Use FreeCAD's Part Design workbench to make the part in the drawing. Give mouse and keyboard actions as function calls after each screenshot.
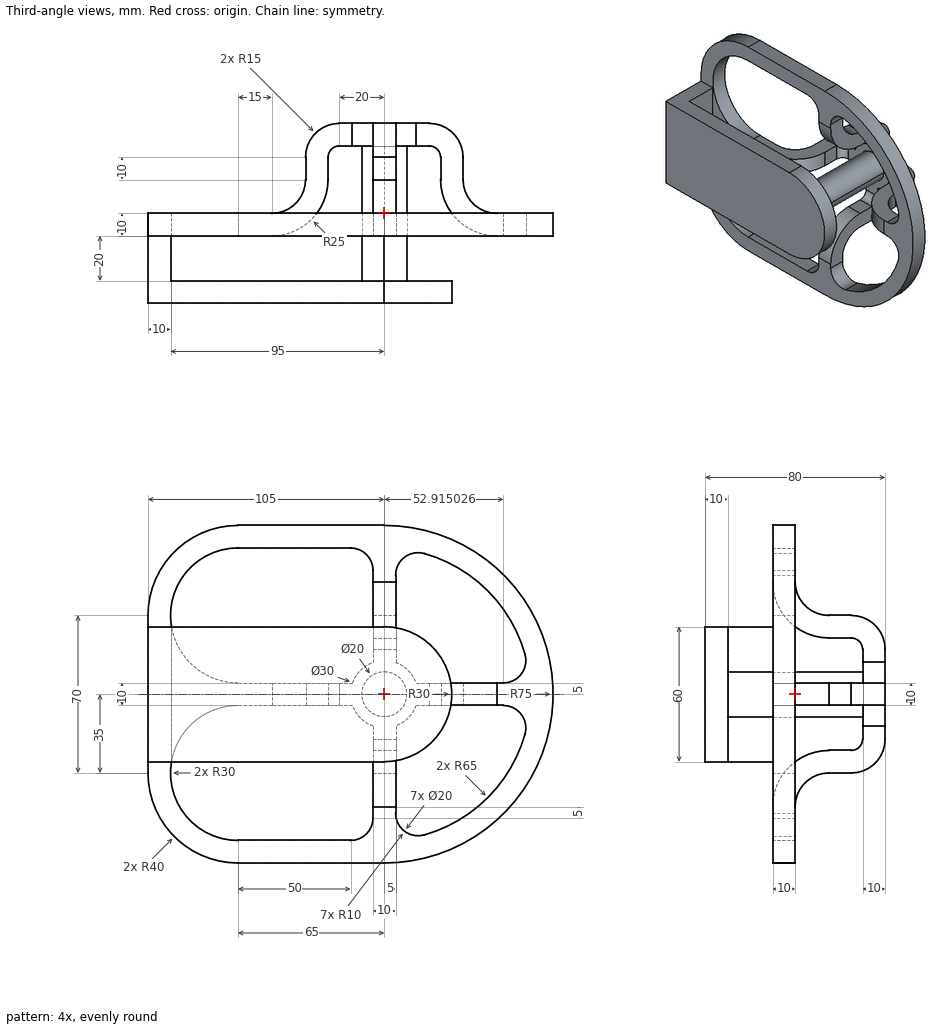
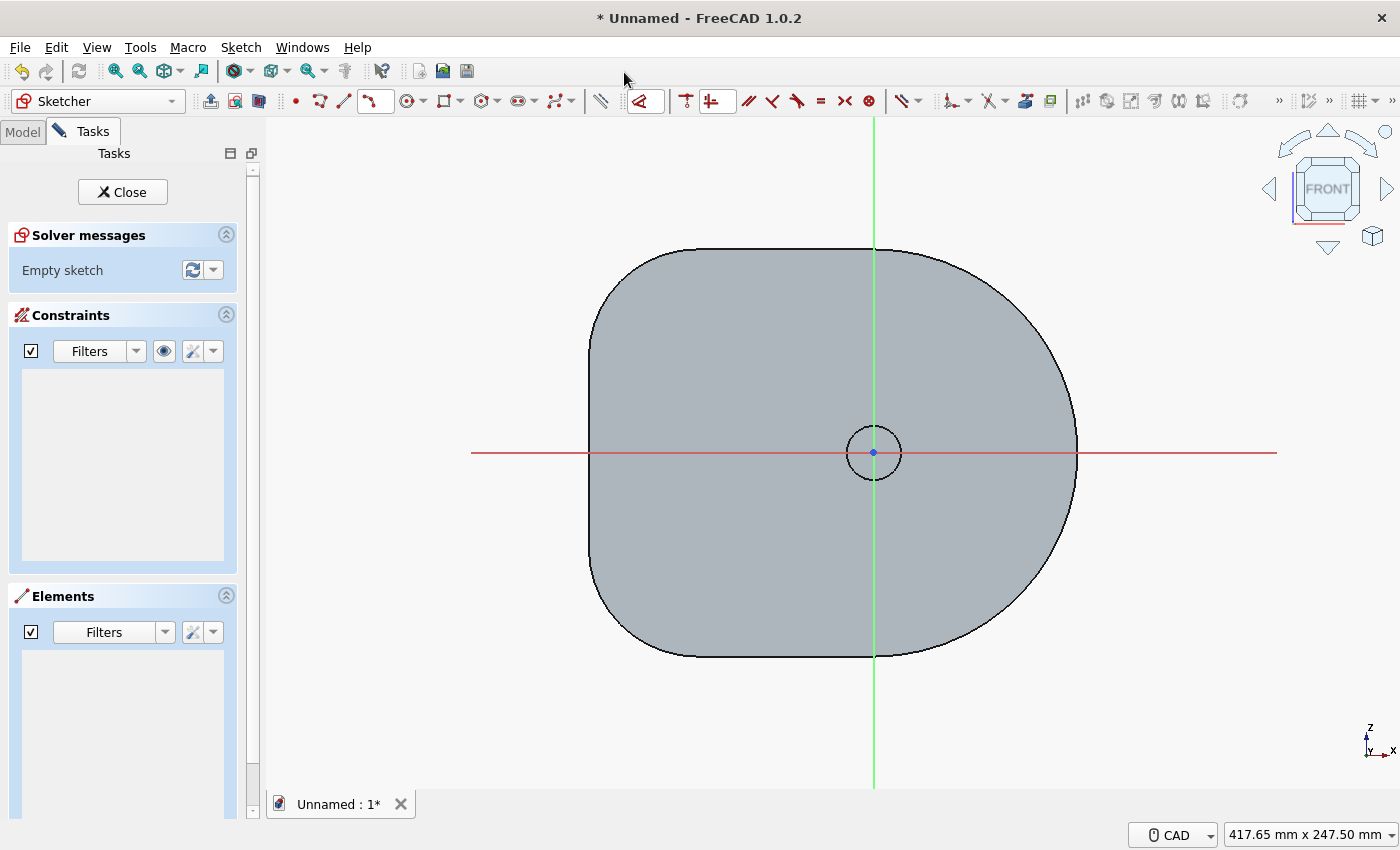
scroll(781, 453, up, 3)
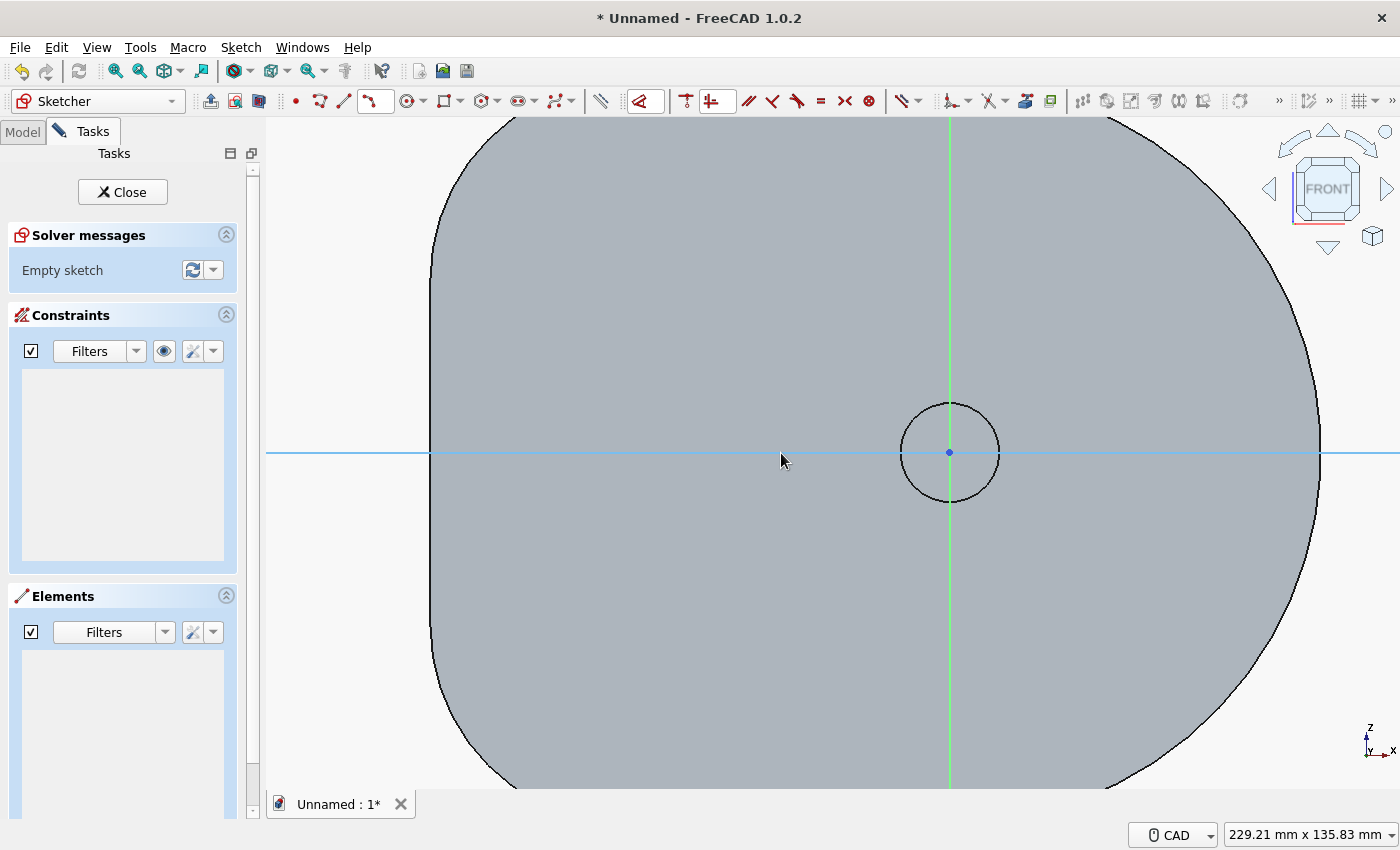
click(320, 102)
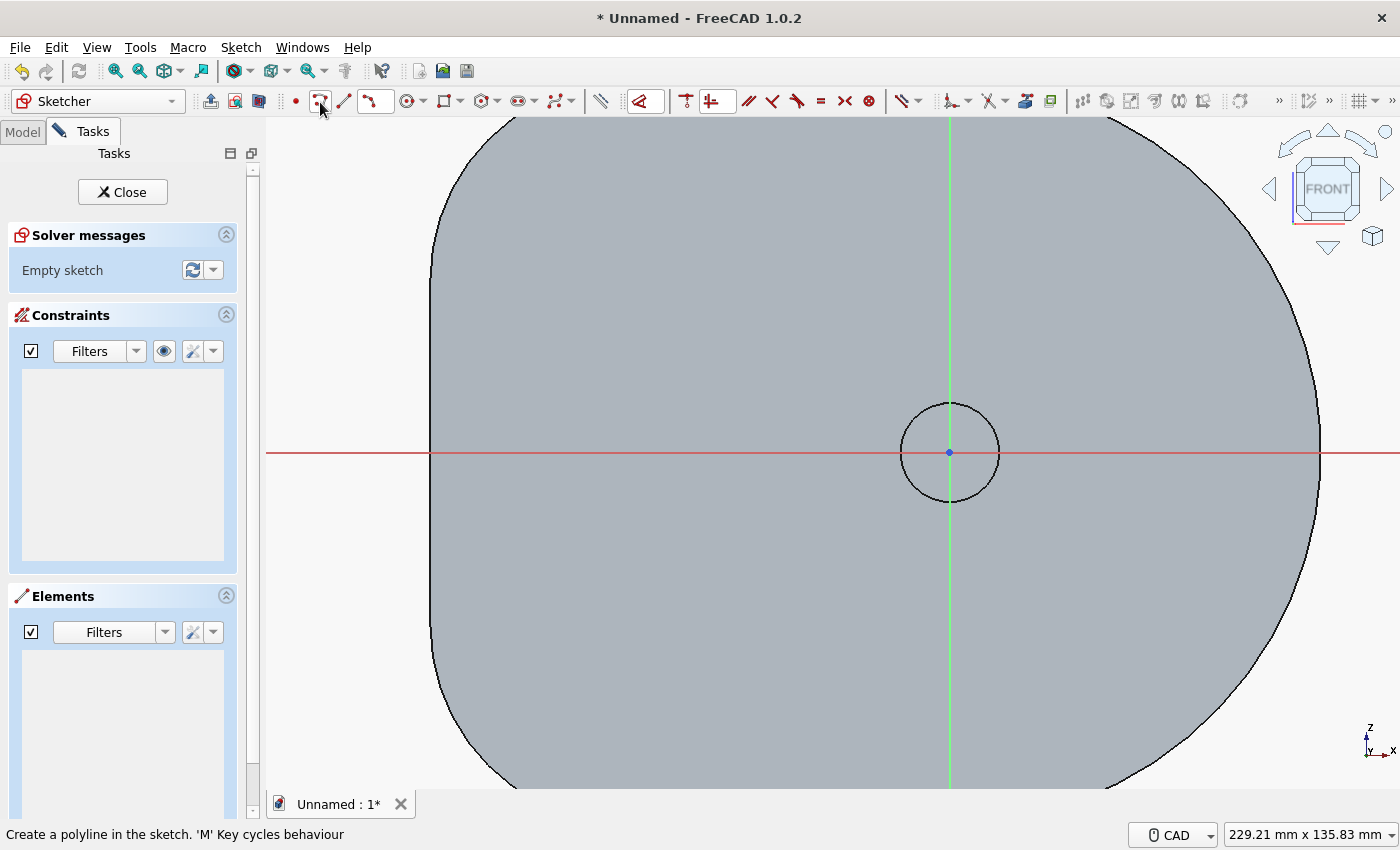
click(950, 304)
click(430, 304)
click(430, 601)
click(950, 601)
right_click(950, 601)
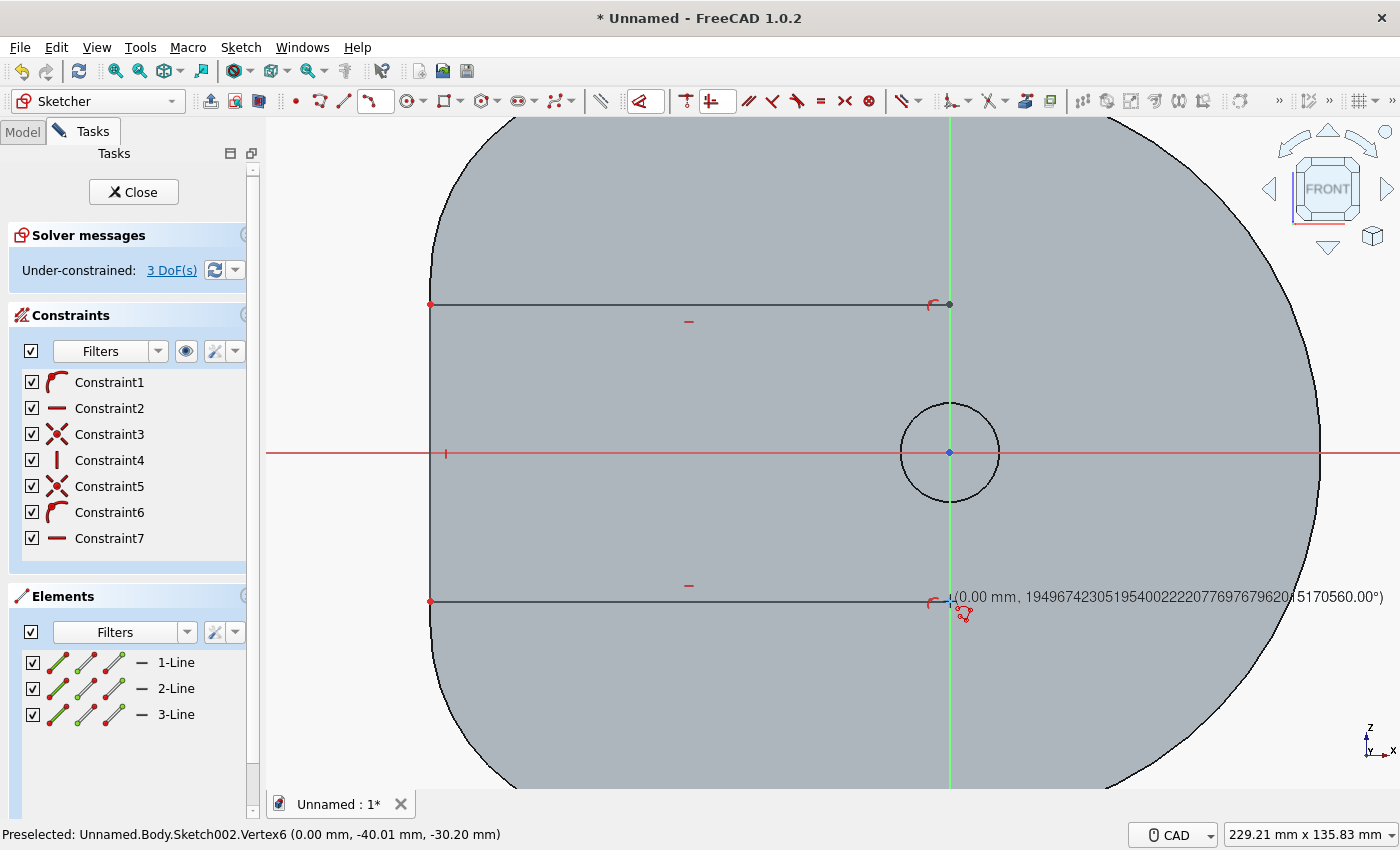
click(370, 102)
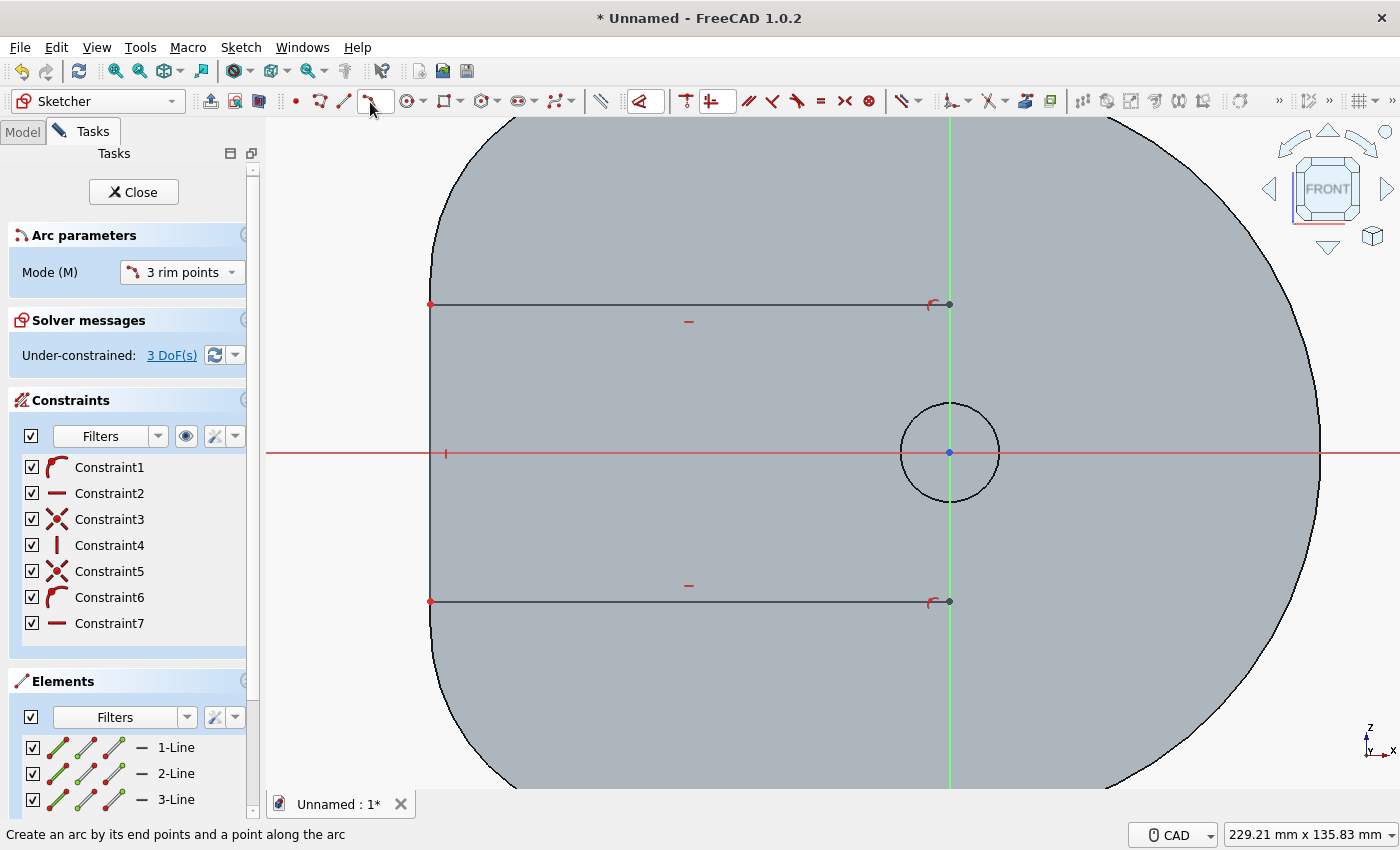
click(950, 602)
click(950, 305)
click(1091, 498)
key(Escape)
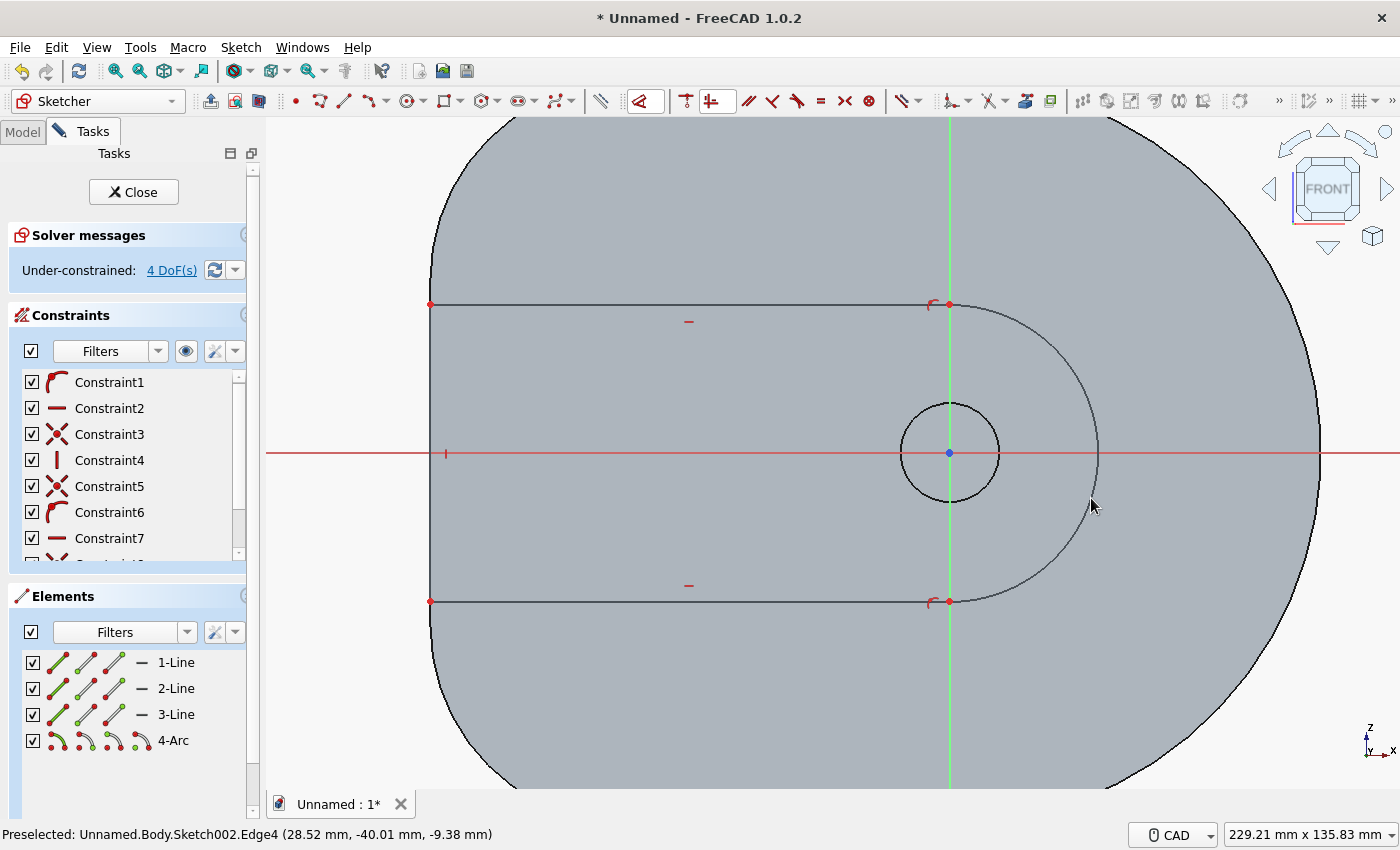
drag(940, 443, 960, 463)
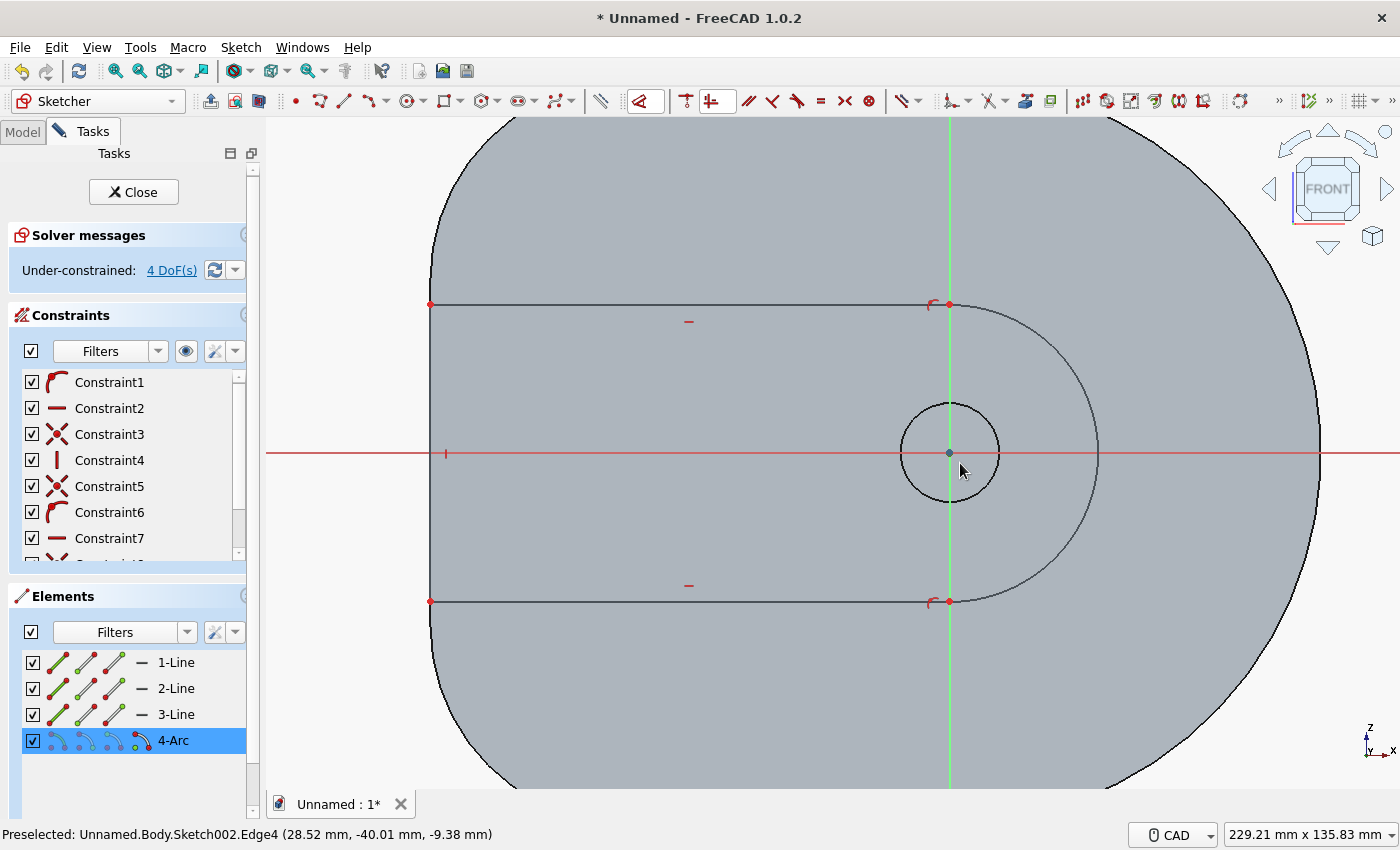
click(686, 102)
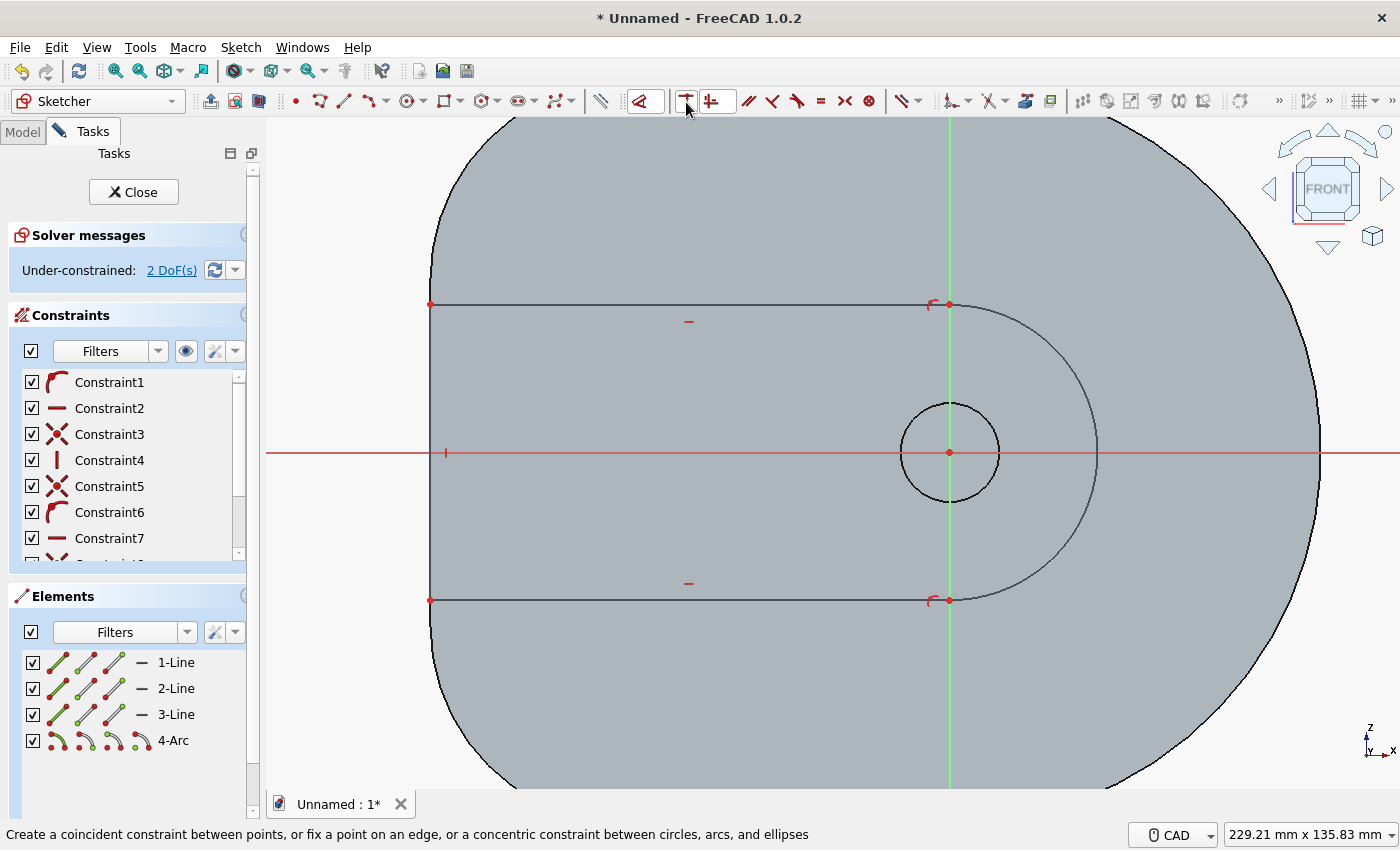
click(1069, 539)